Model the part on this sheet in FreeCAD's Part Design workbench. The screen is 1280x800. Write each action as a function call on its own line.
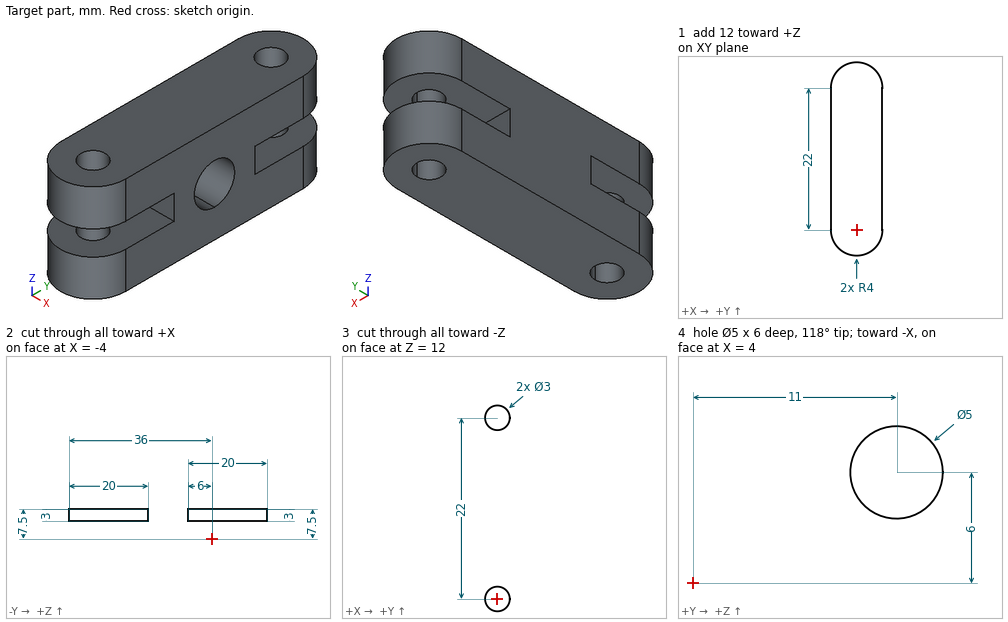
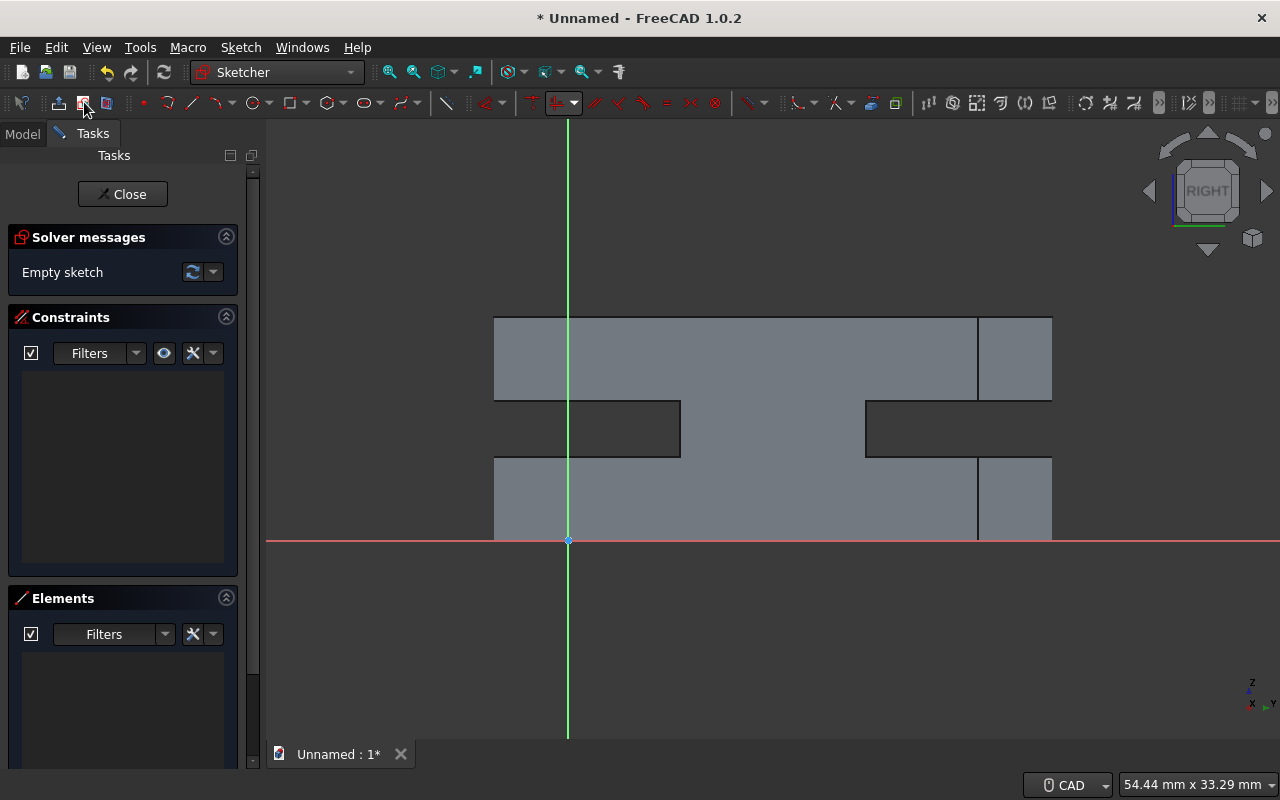
scroll(795, 429, up, 7)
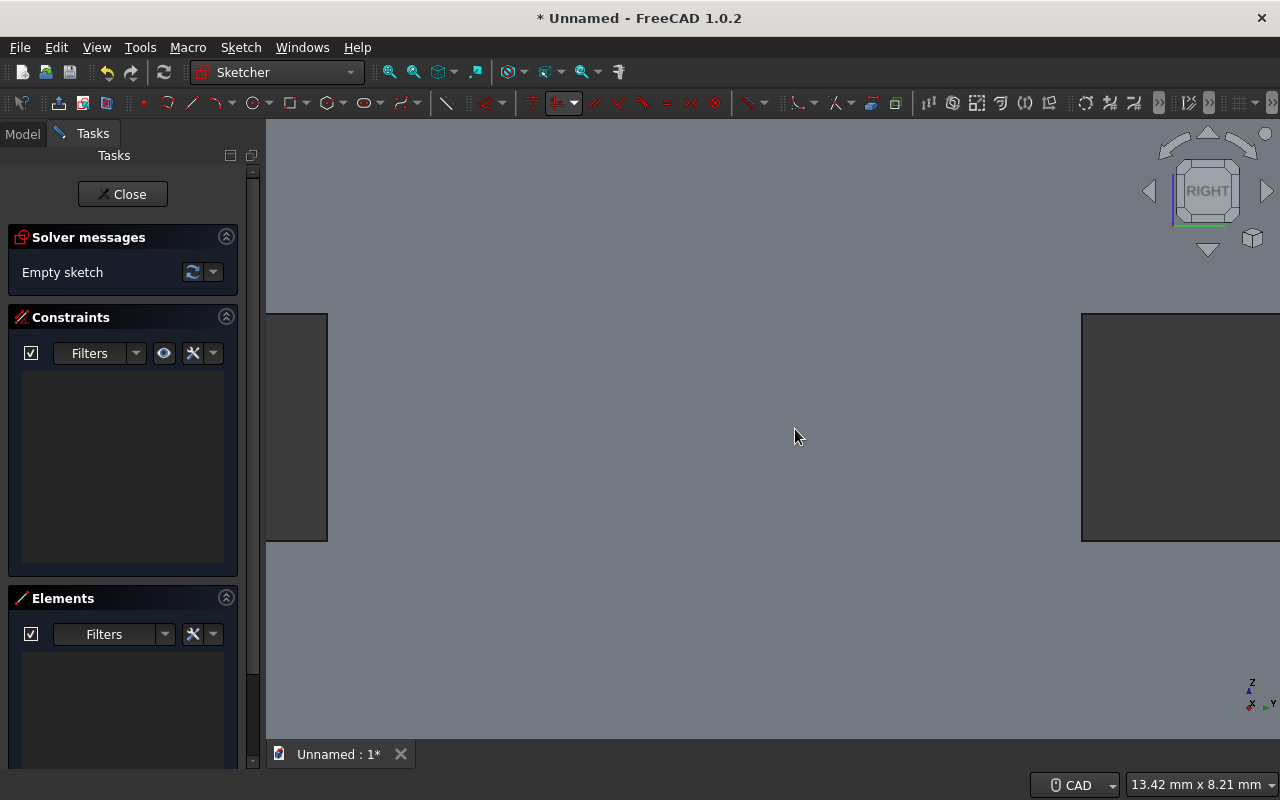
key(g)
key(c)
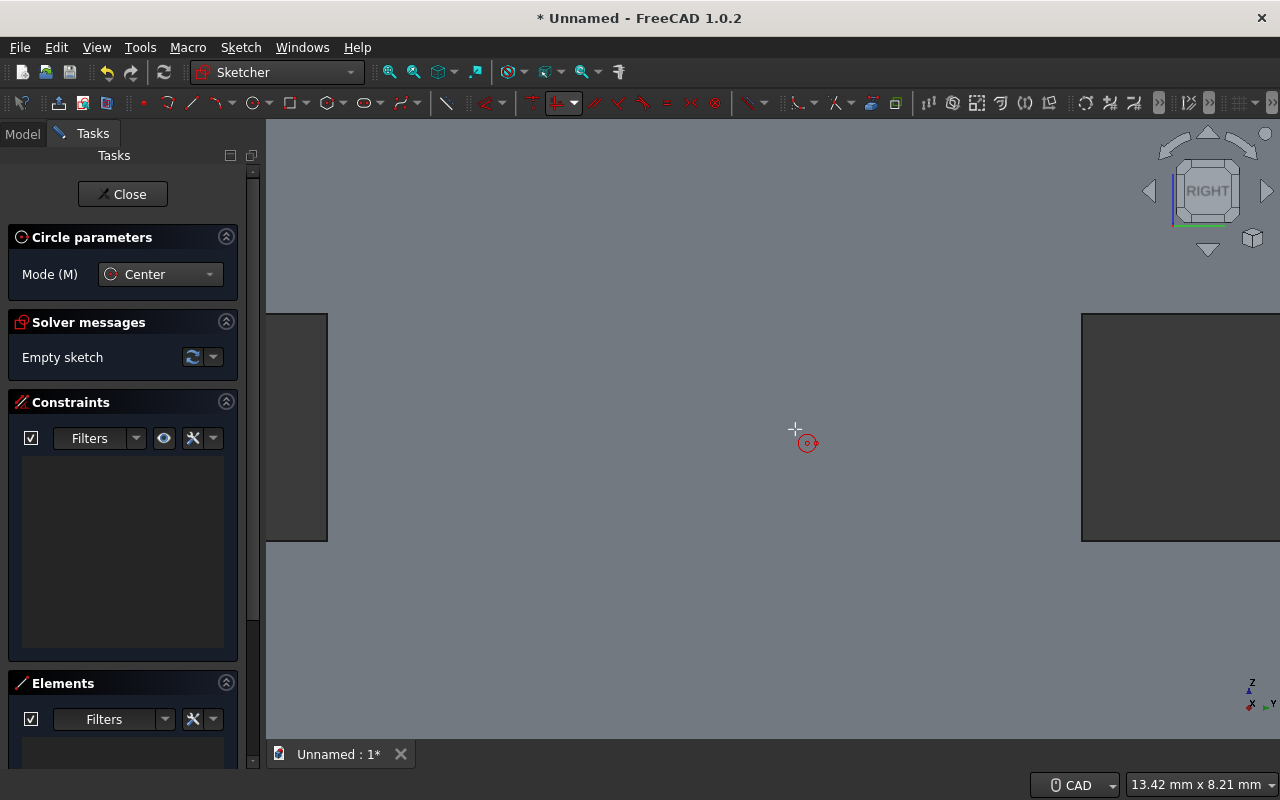
click(704, 427)
move(838, 294)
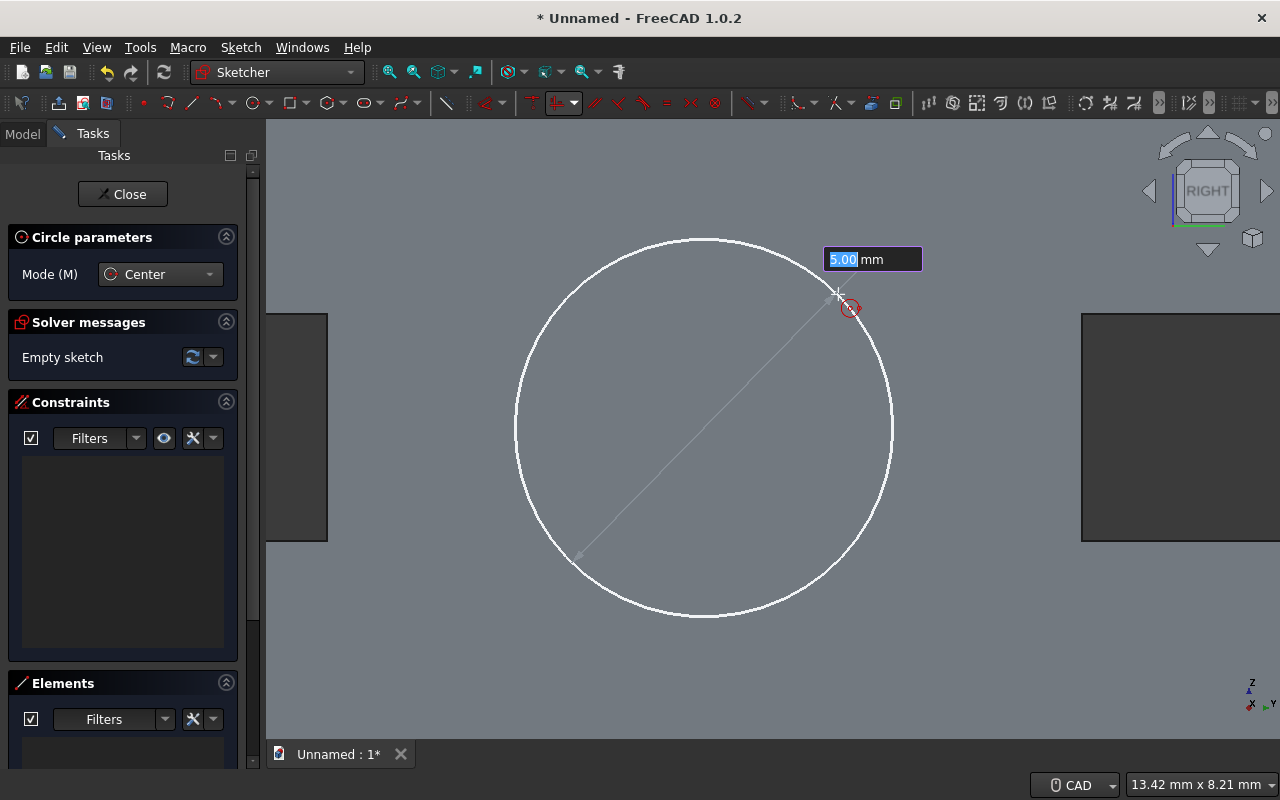
text(5)
key(Return)
key(Escape)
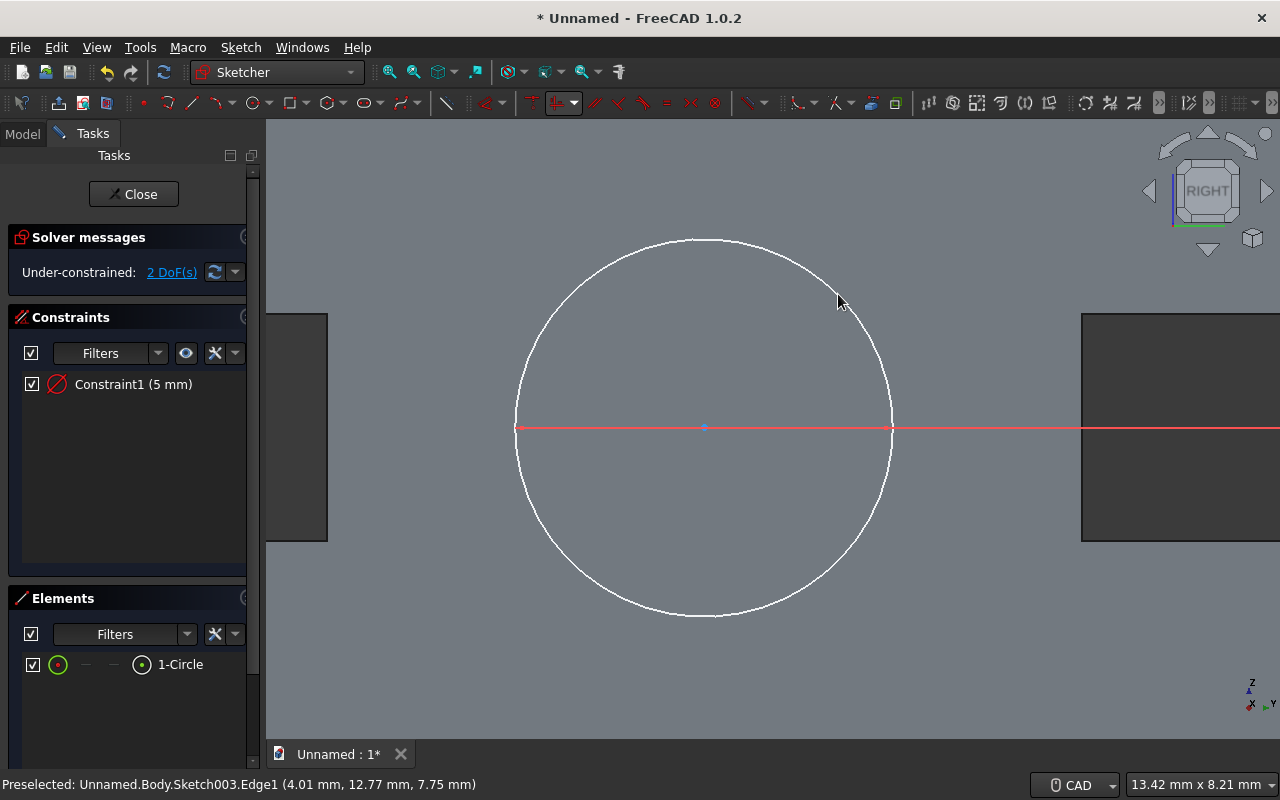
key(d)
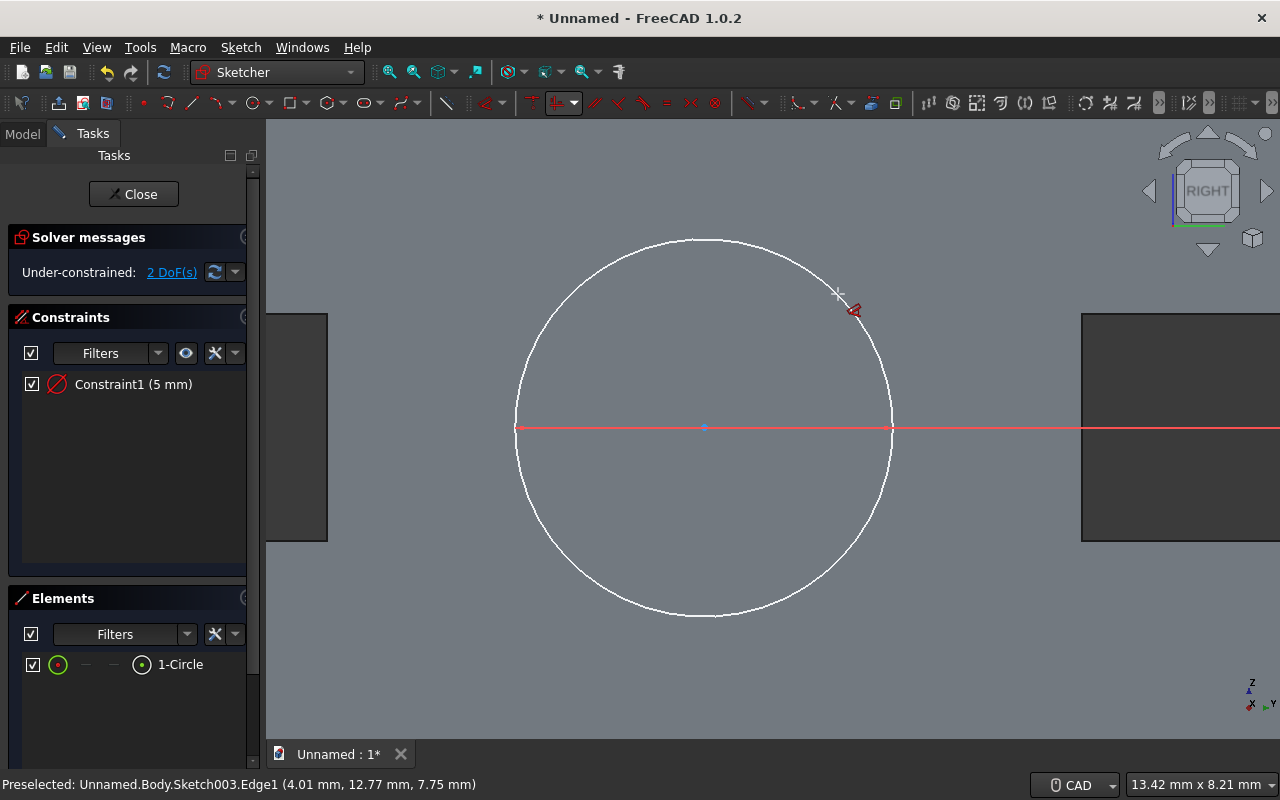
click(704, 428)
click(738, 569)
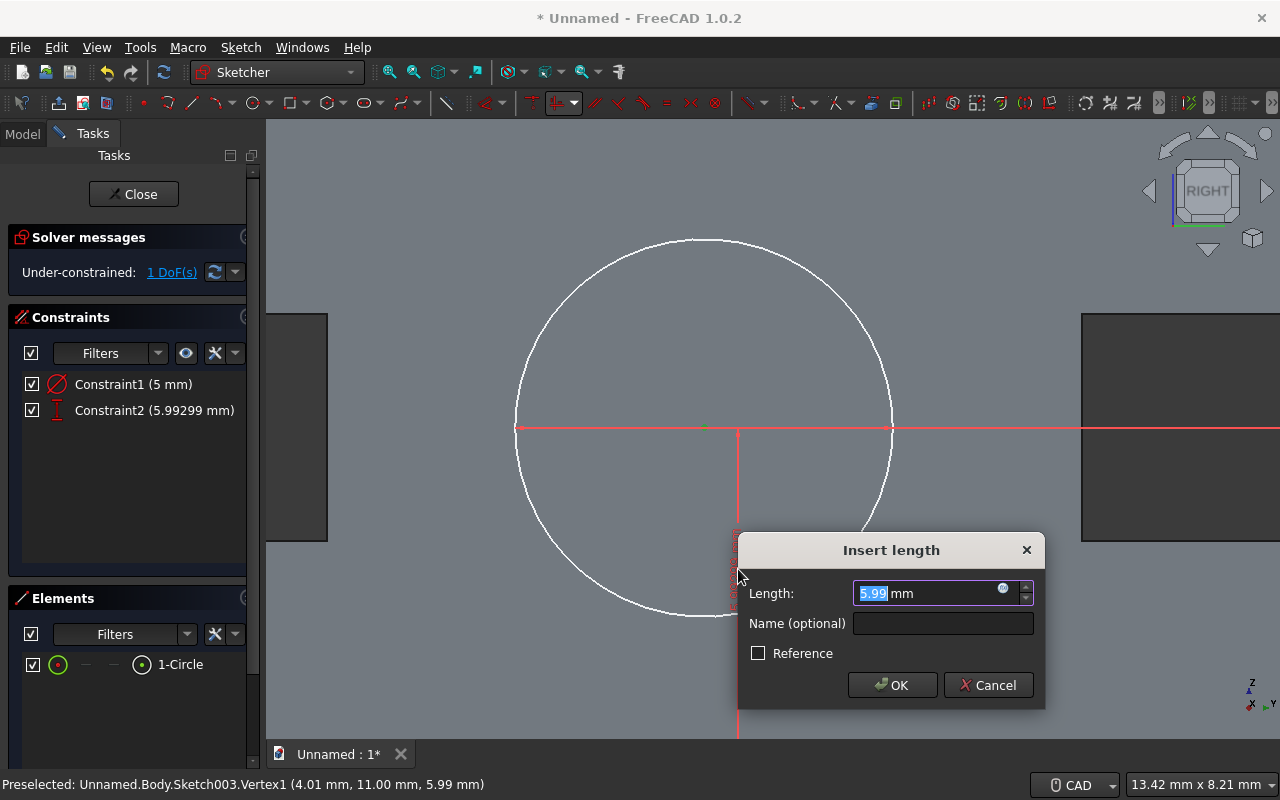
text(6)
key(Return)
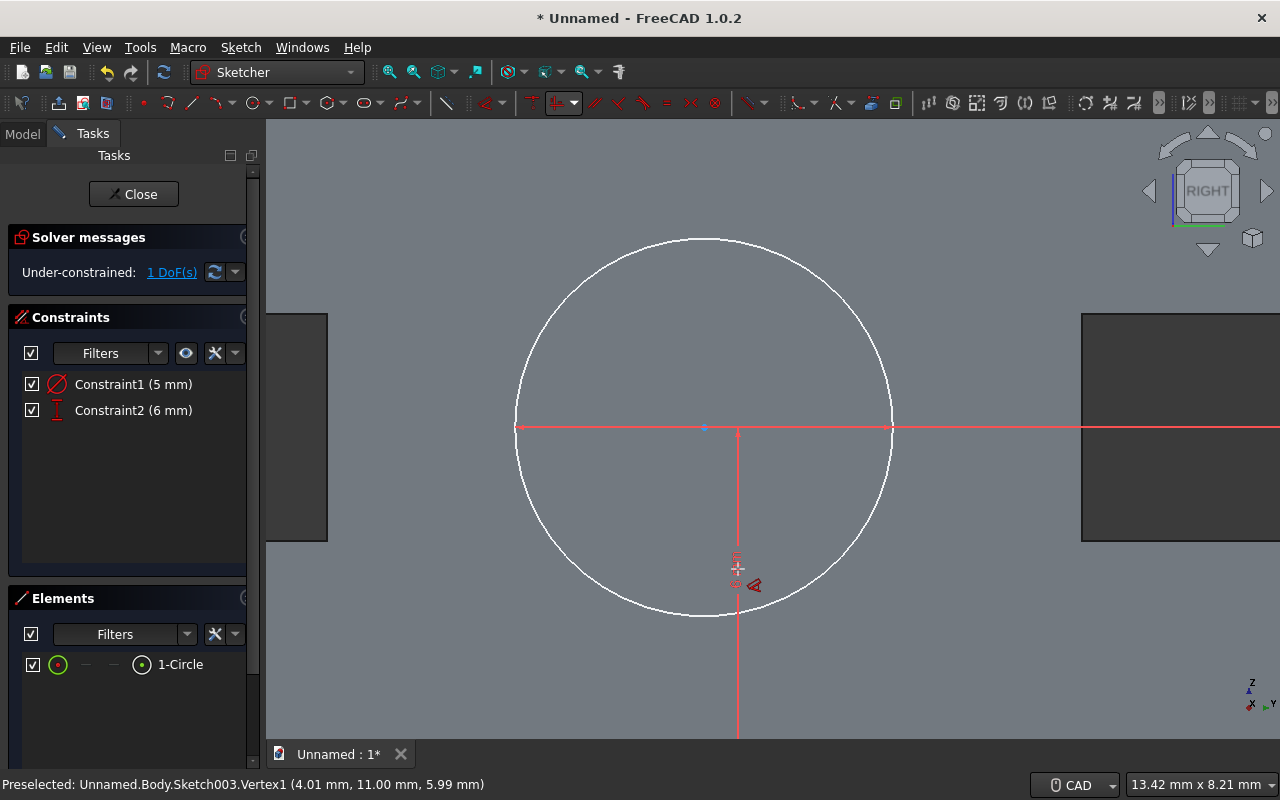
click(704, 427)
click(499, 393)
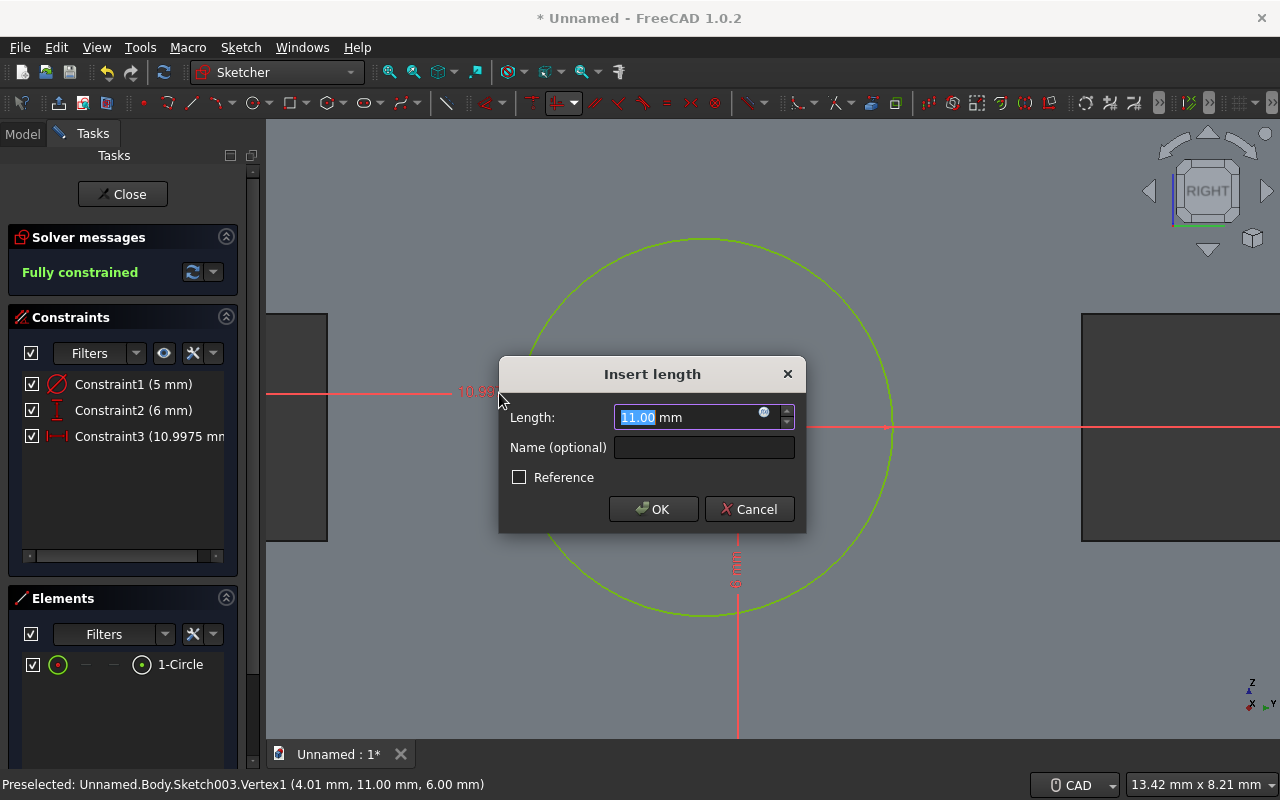
text(11)
key(Return)
key(Escape)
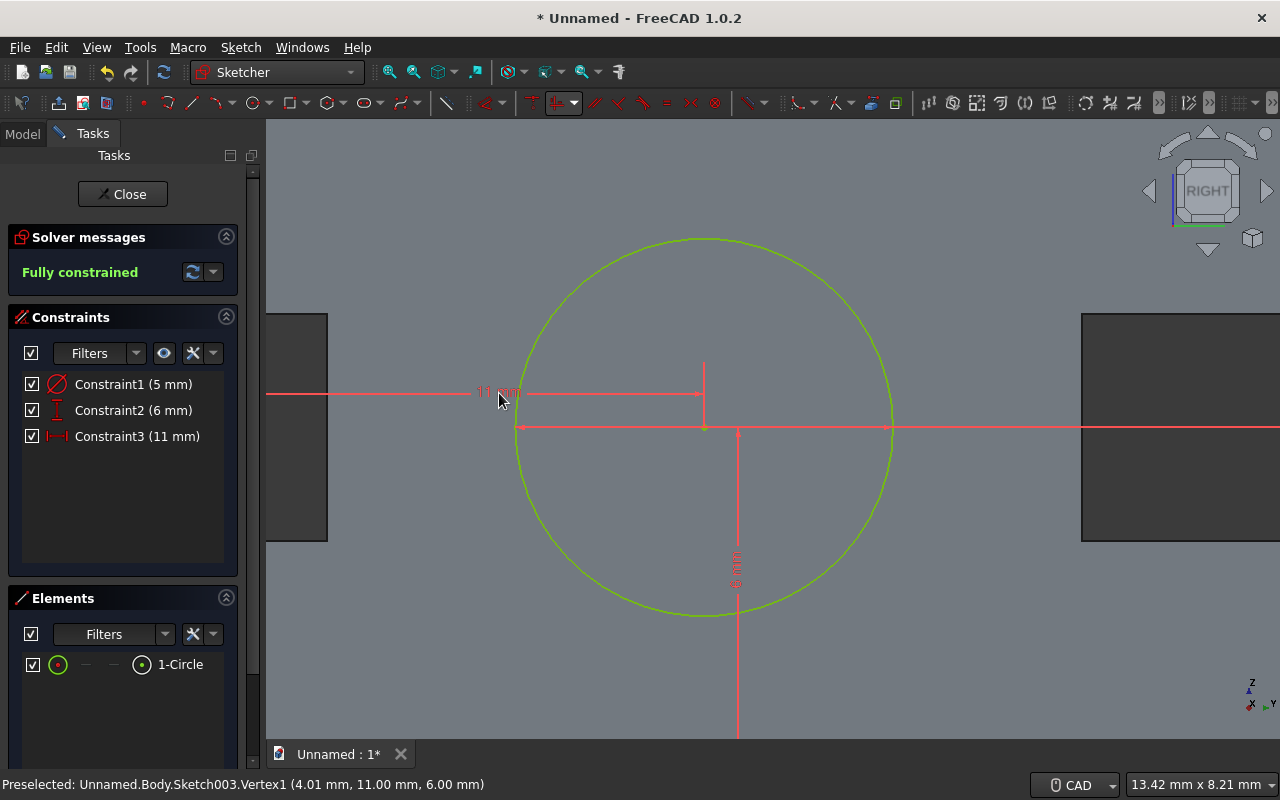
click(123, 194)